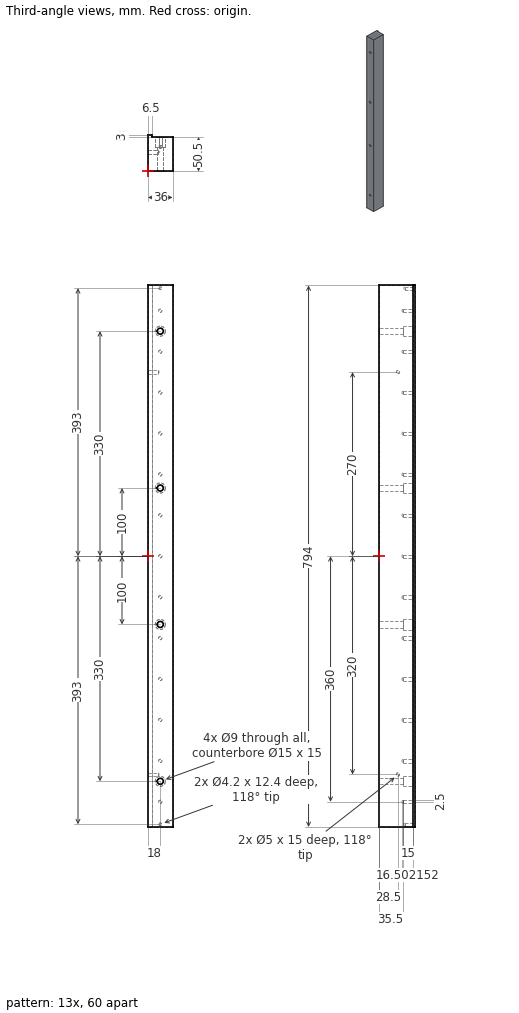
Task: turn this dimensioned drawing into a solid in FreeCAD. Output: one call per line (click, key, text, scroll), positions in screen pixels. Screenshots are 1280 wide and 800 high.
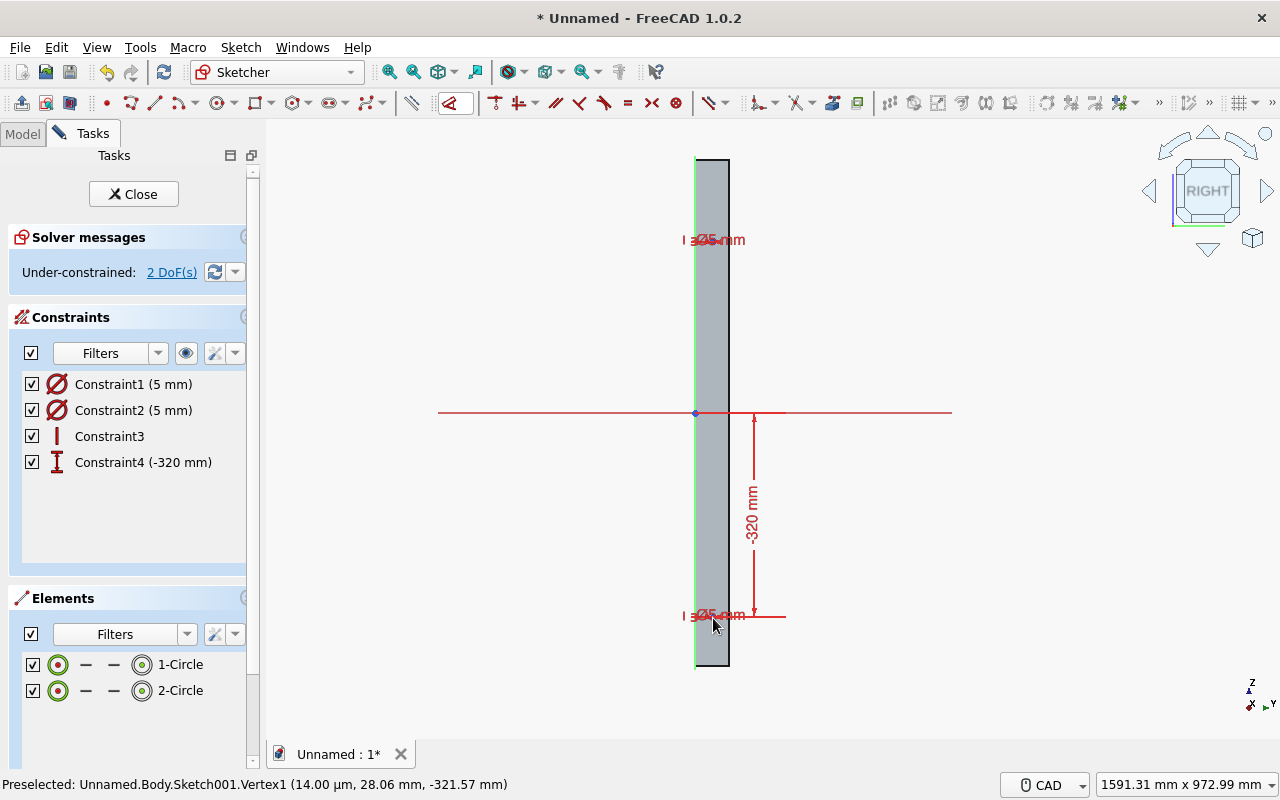
click(713, 242)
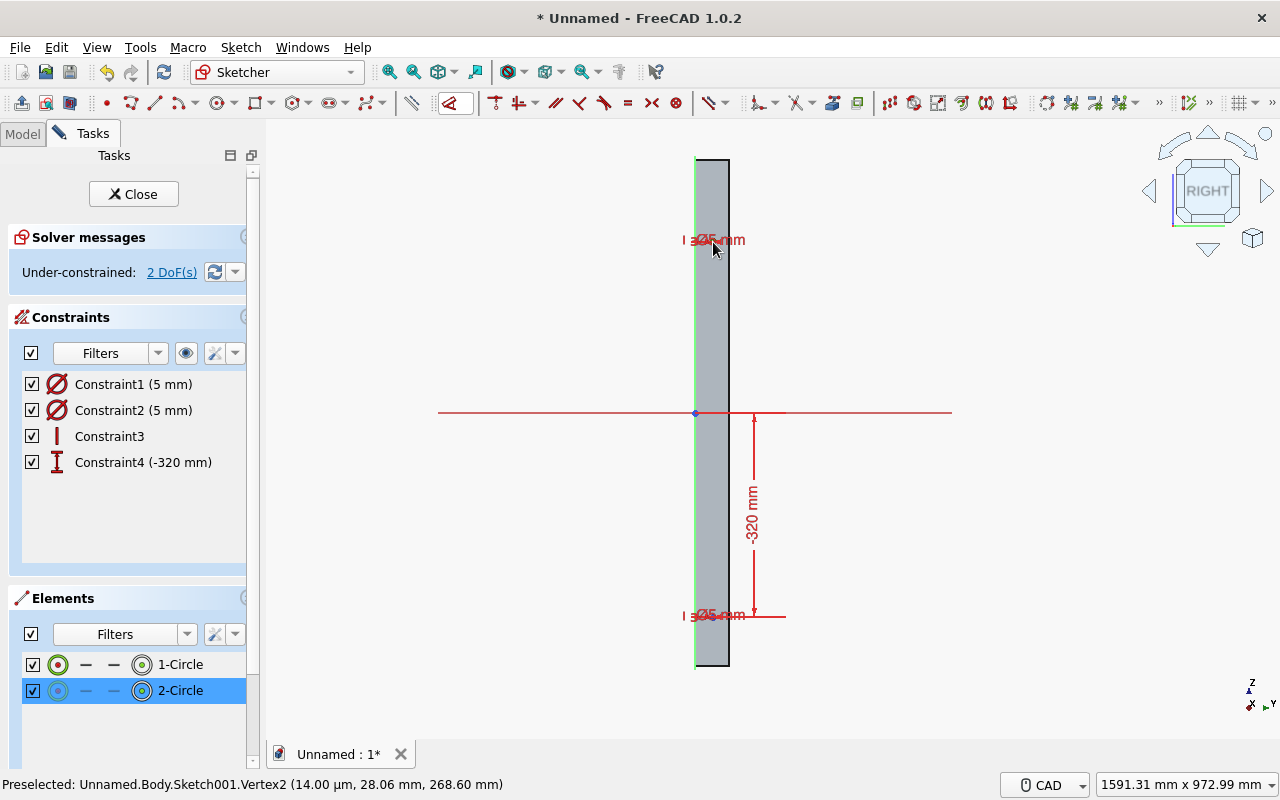
click(468, 104)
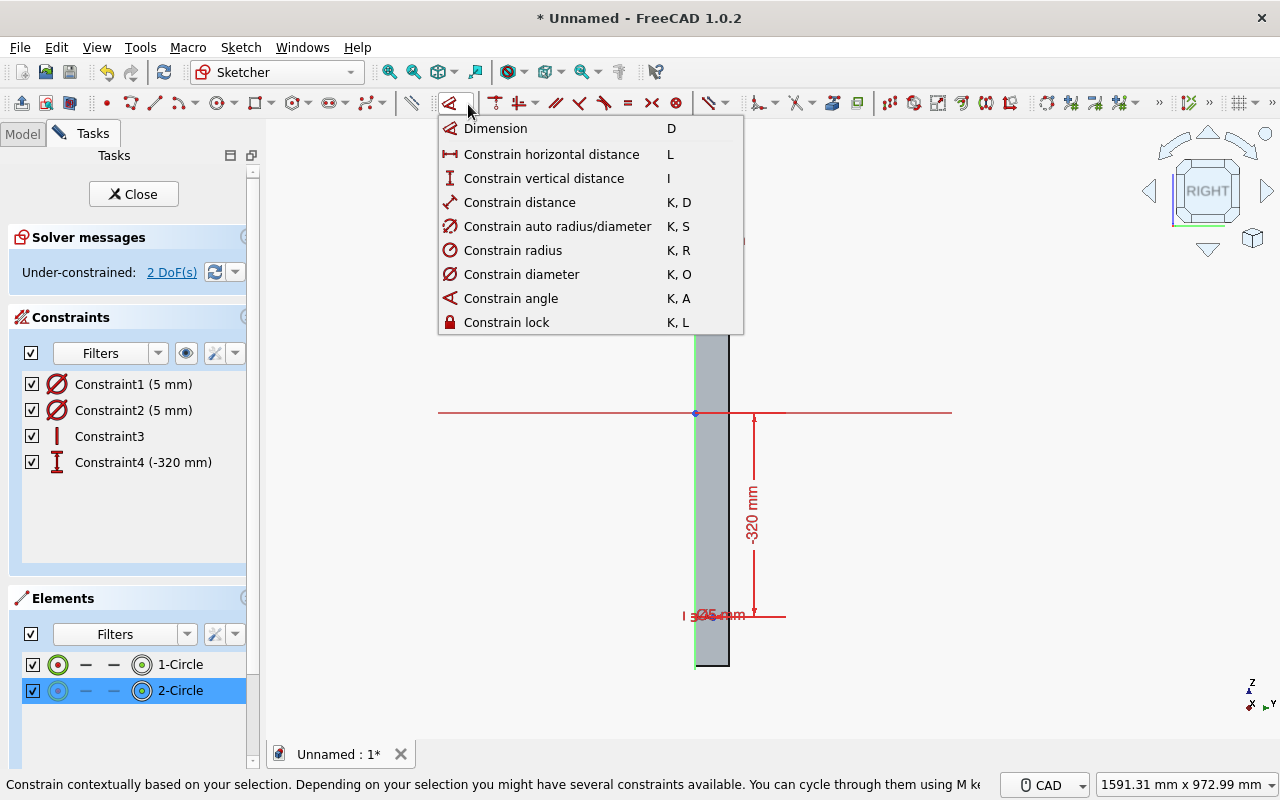
click(591, 178)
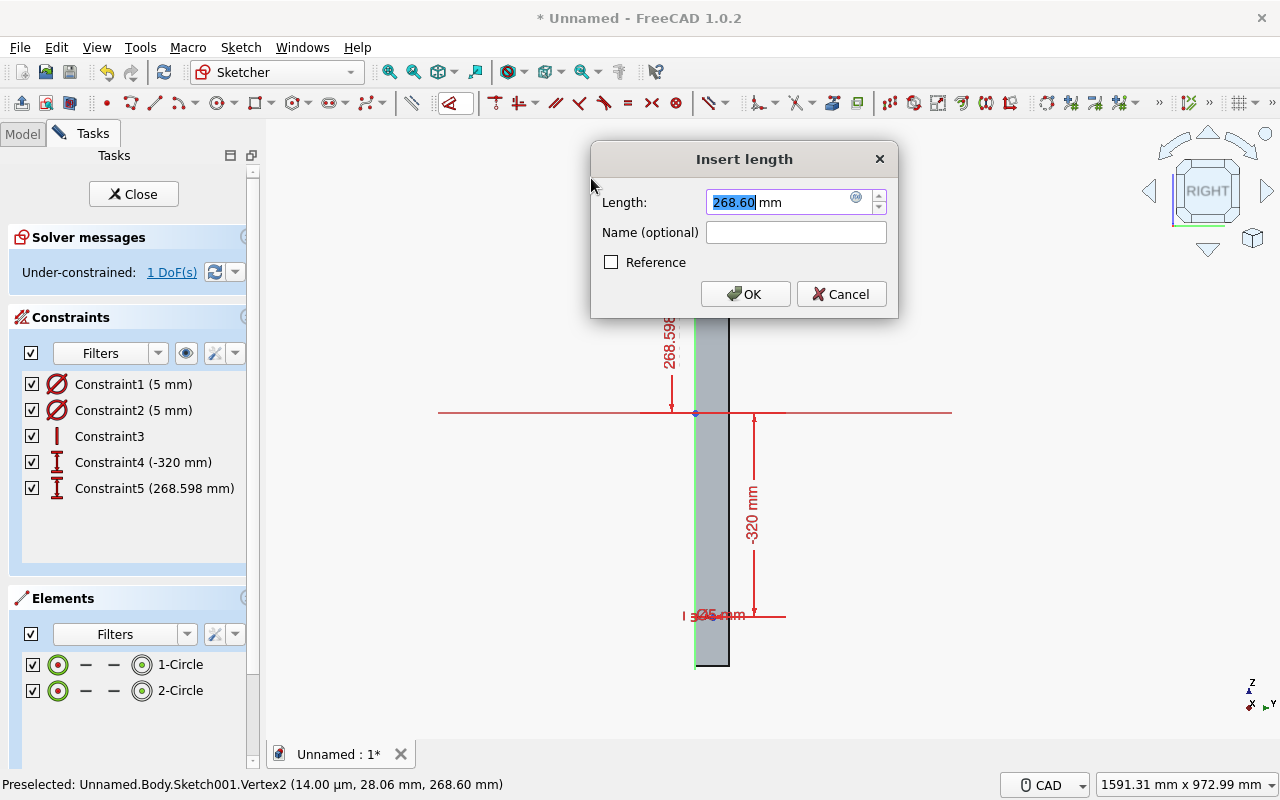
text(270)
key(Return)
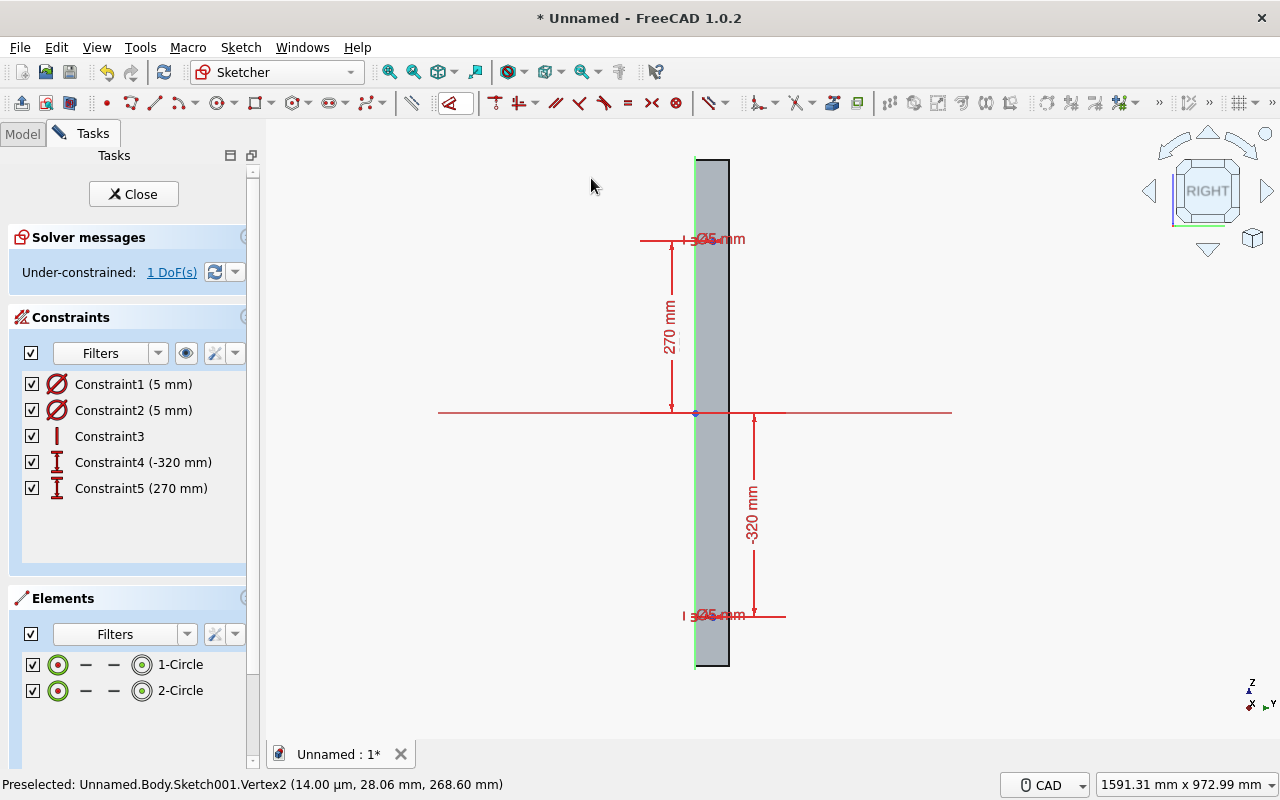
scroll(713, 617, up, 4)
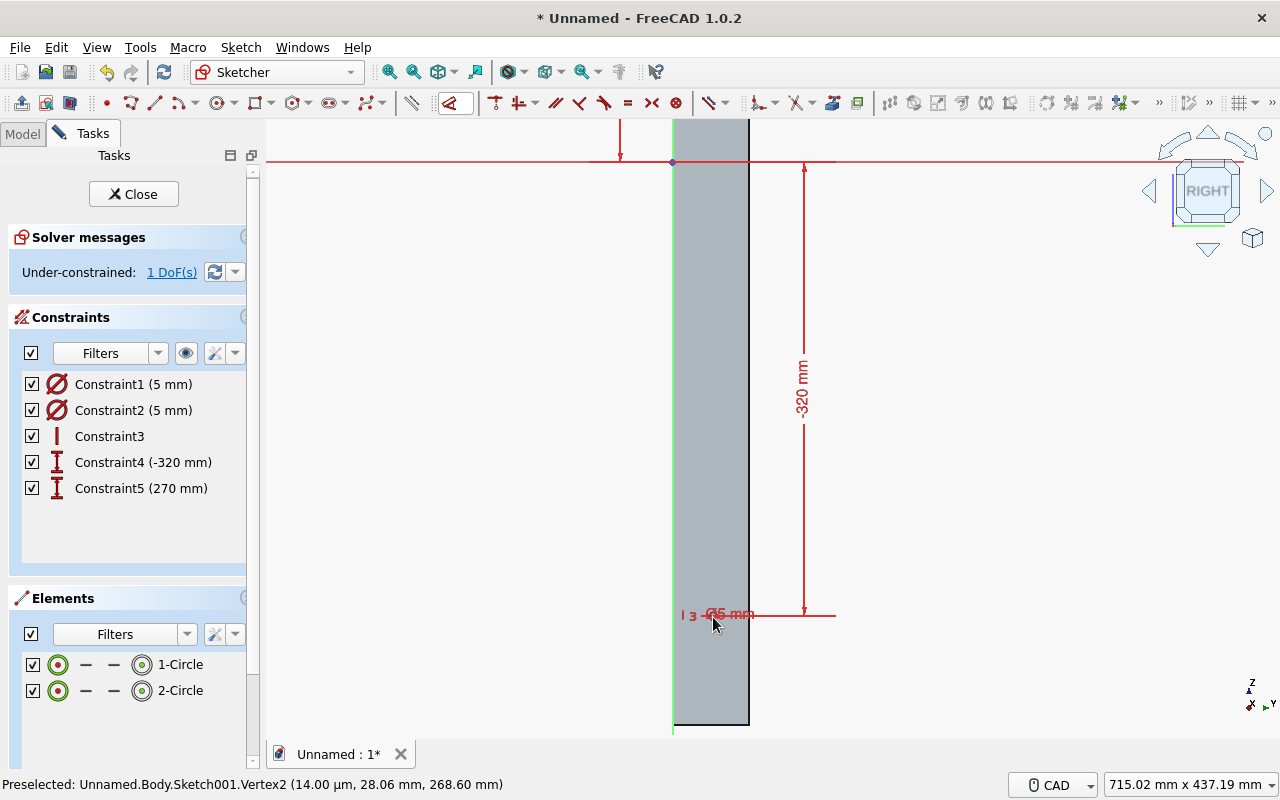
click(712, 616)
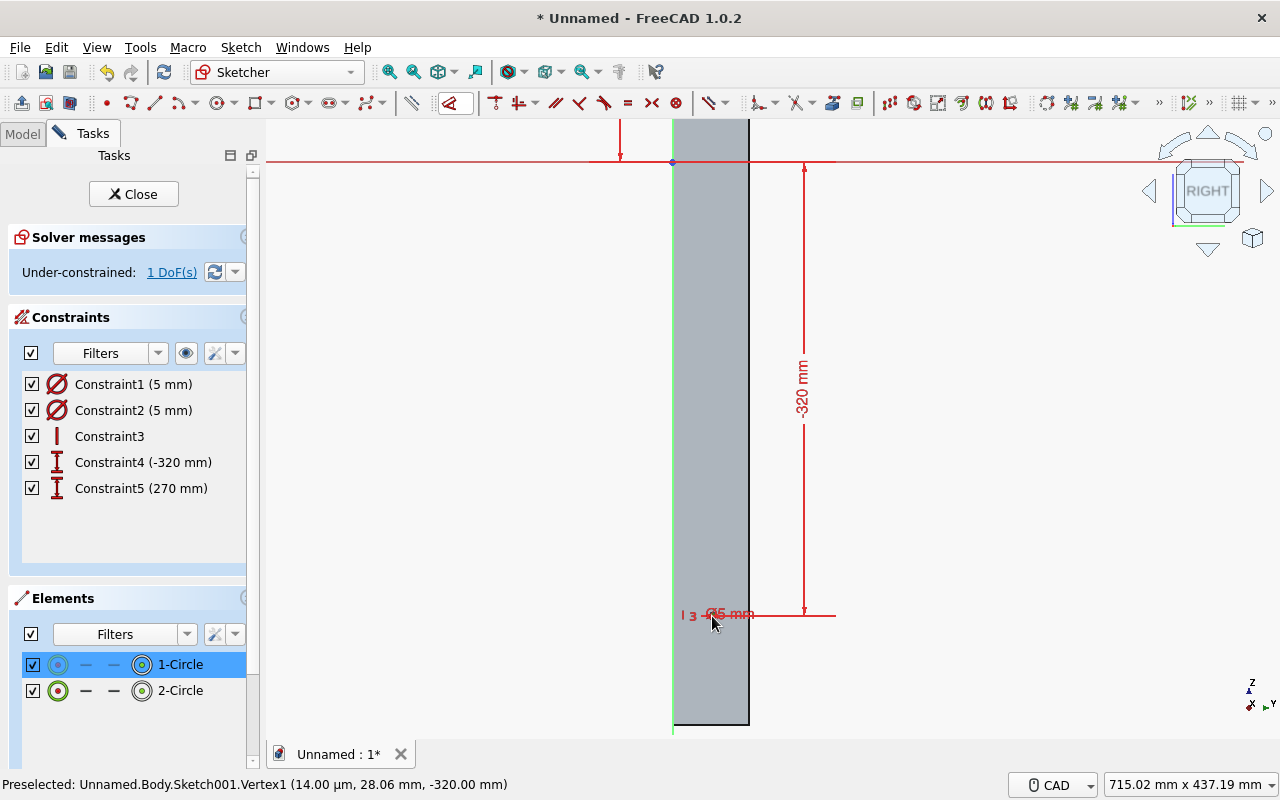
click(468, 104)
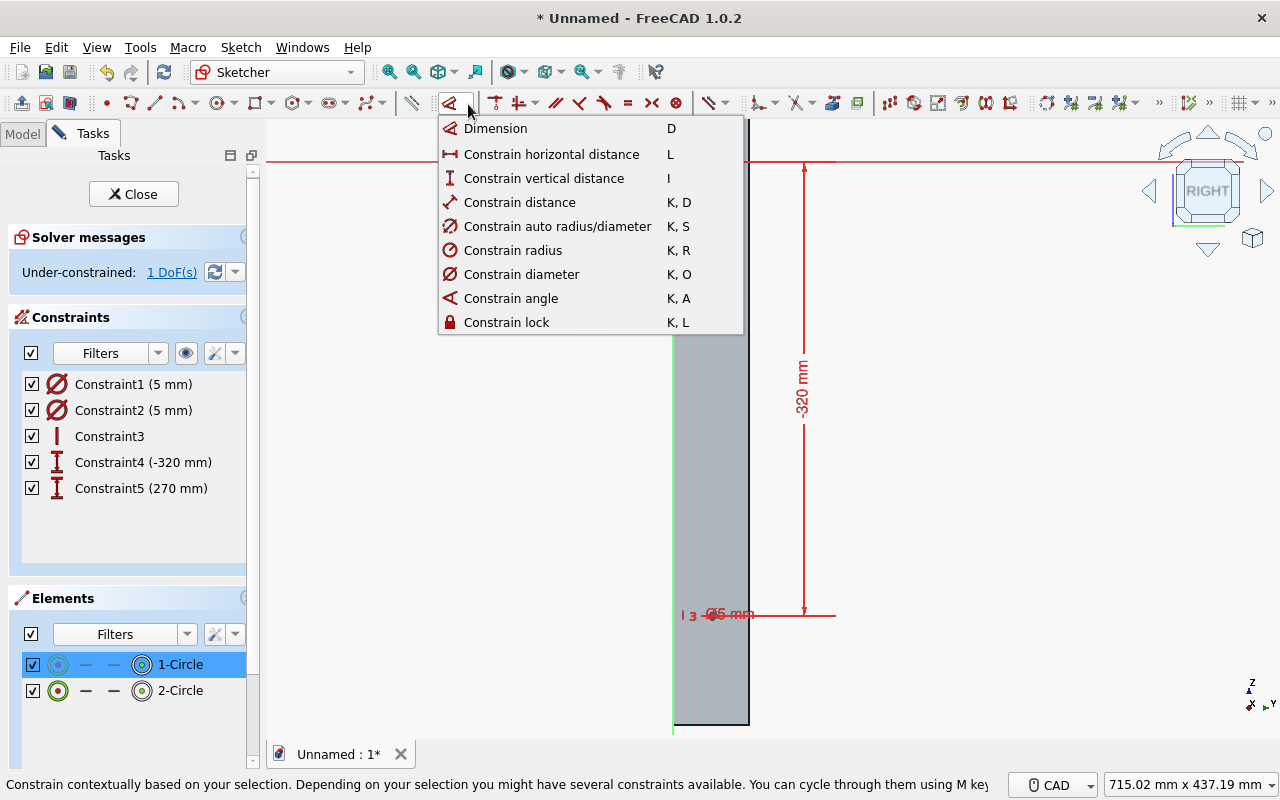
click(591, 154)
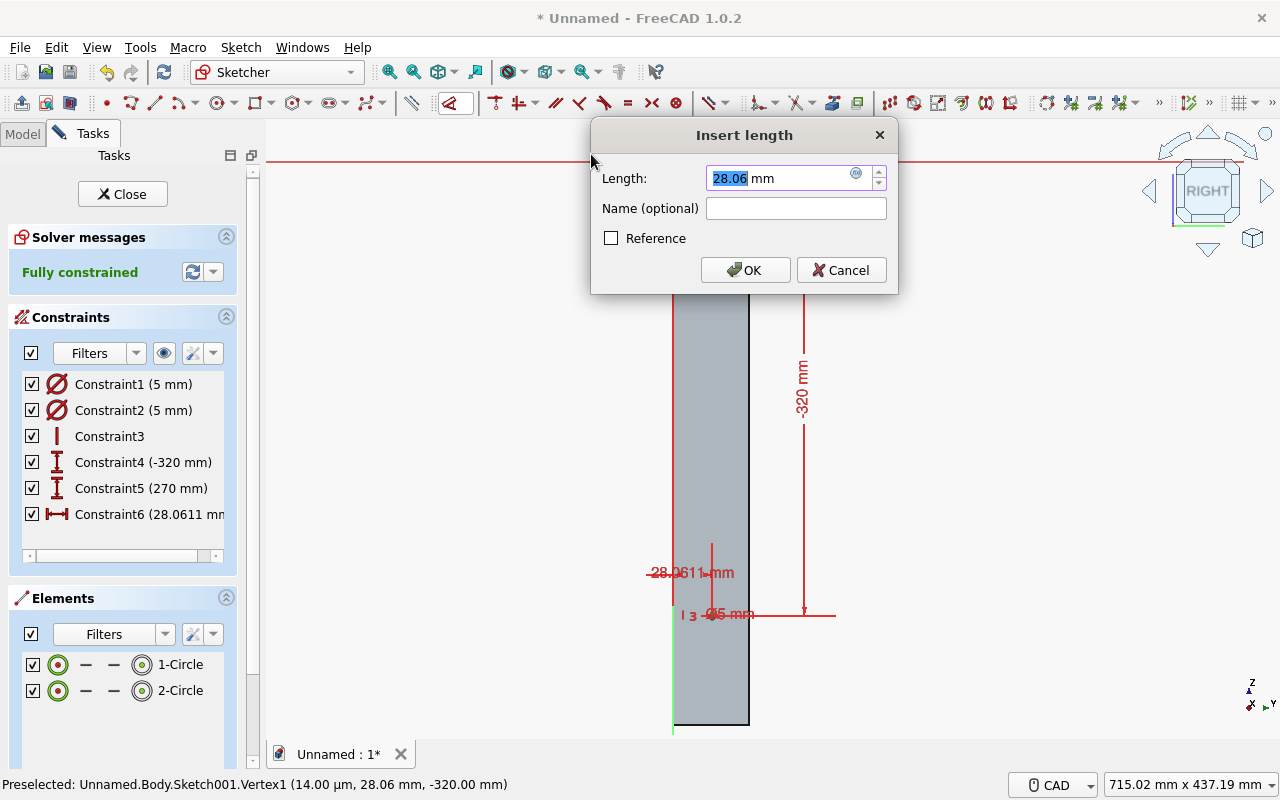
text(28.5)
key(Return)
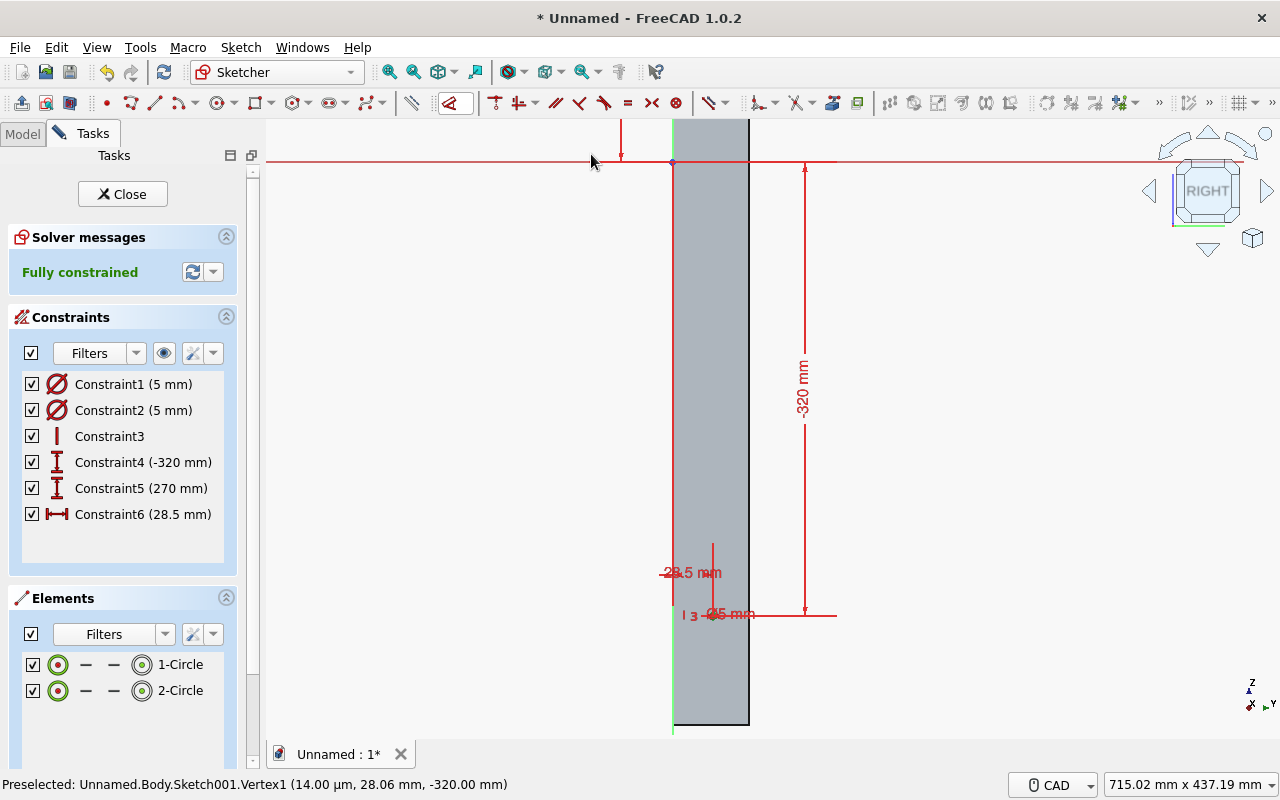
click(123, 194)